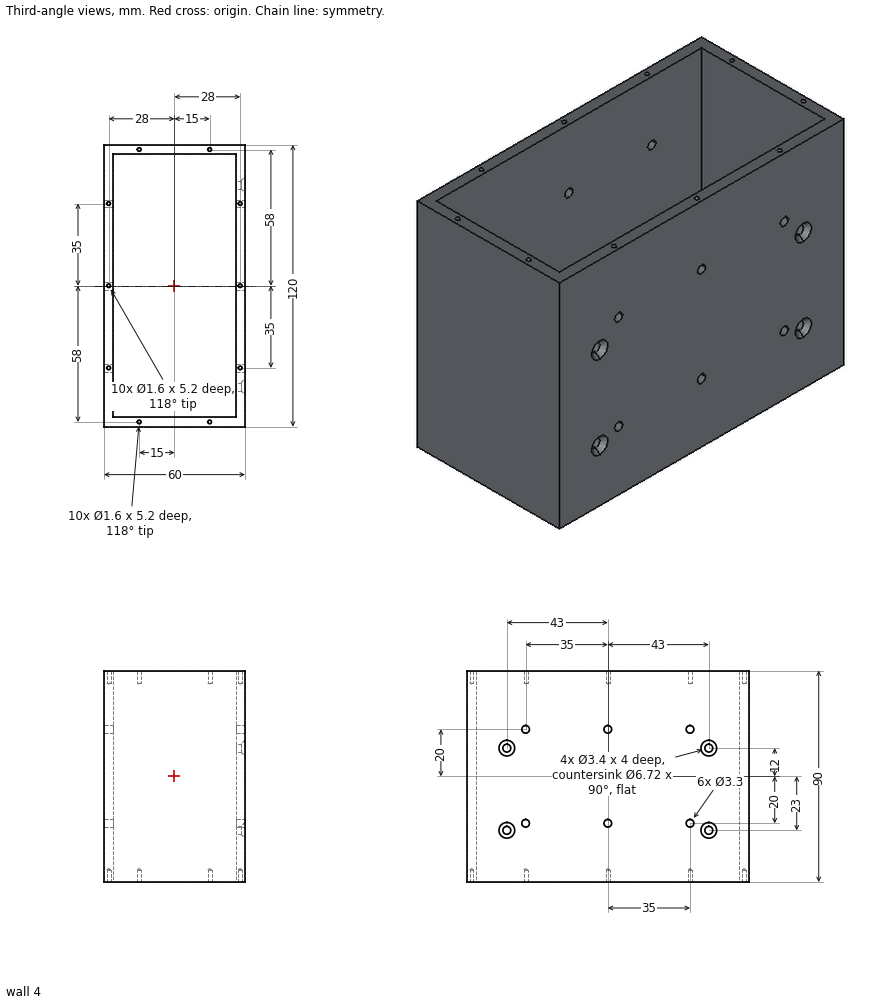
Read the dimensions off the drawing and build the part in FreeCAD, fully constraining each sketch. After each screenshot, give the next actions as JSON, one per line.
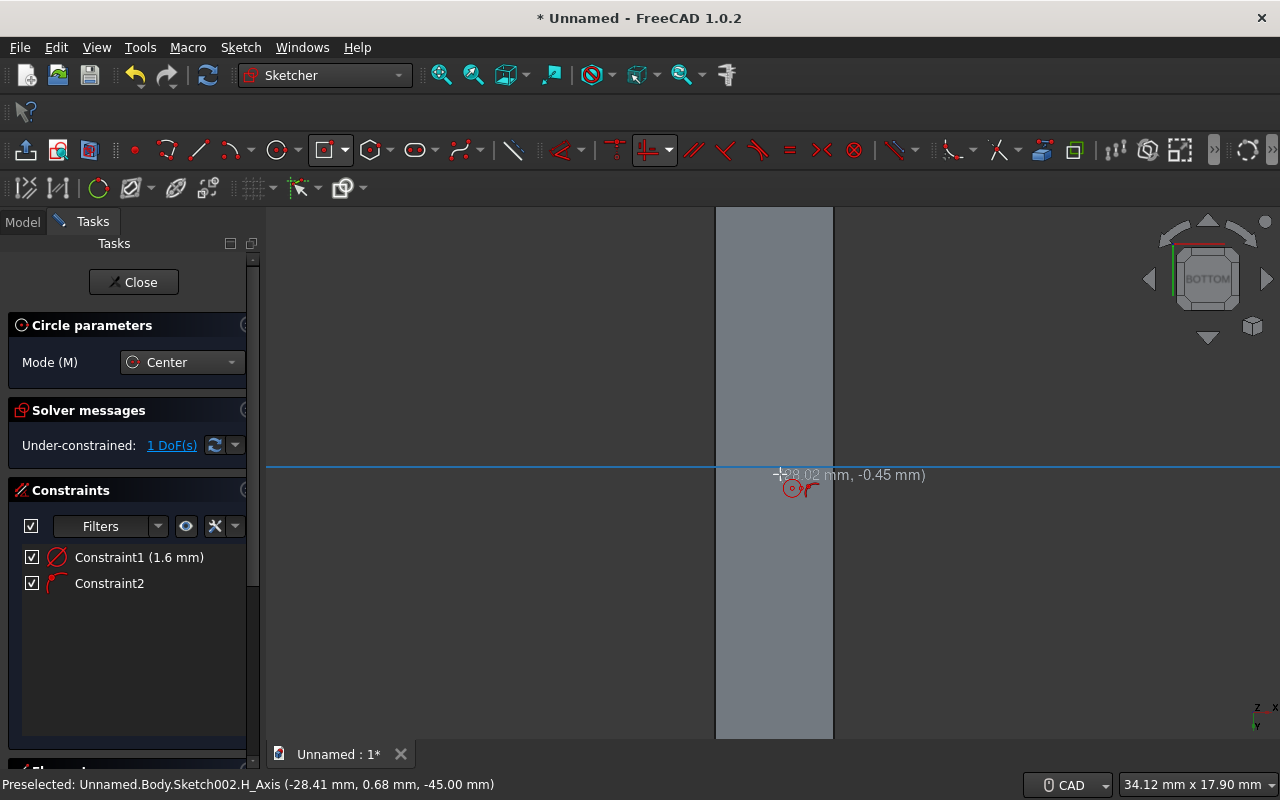
{"action": "scroll", "coordinate": [781, 474], "scroll_direction": "down", "scroll_amount": 12}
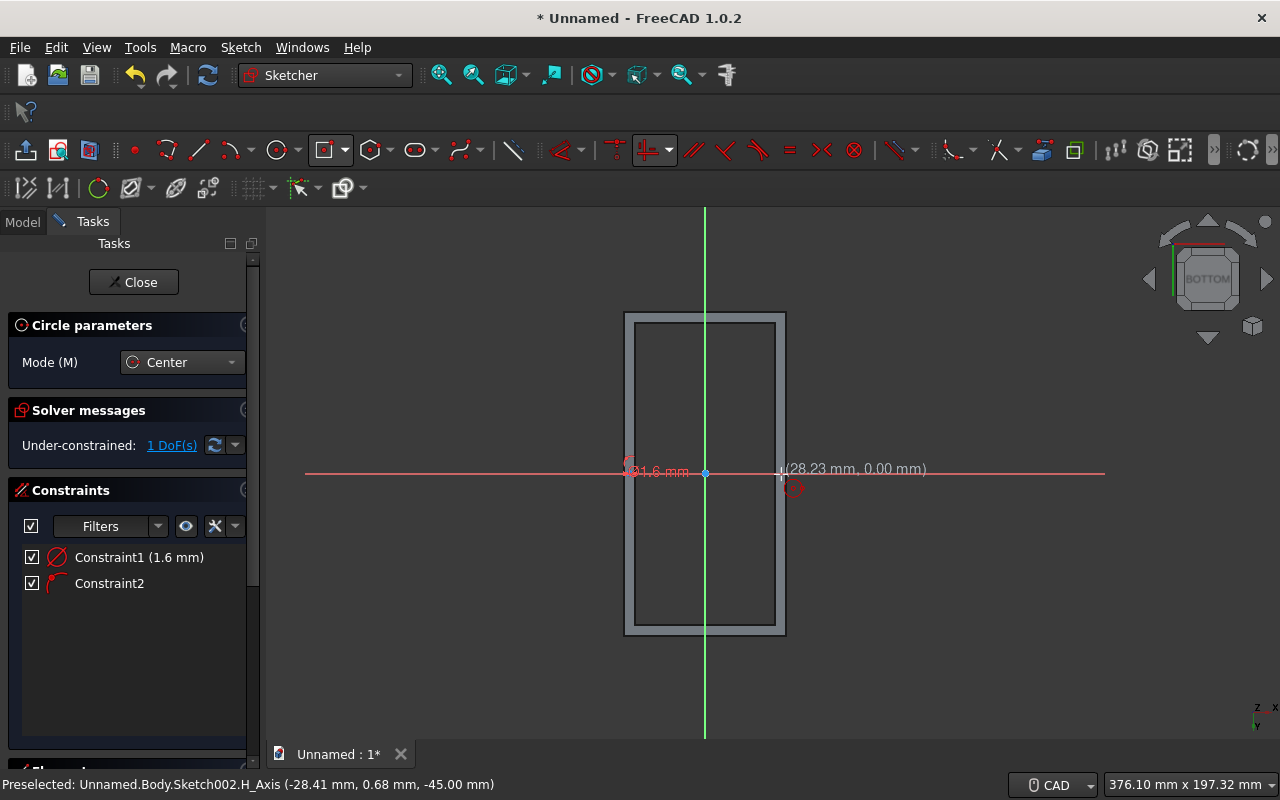
{"action": "left_click", "coordinate": [781, 474]}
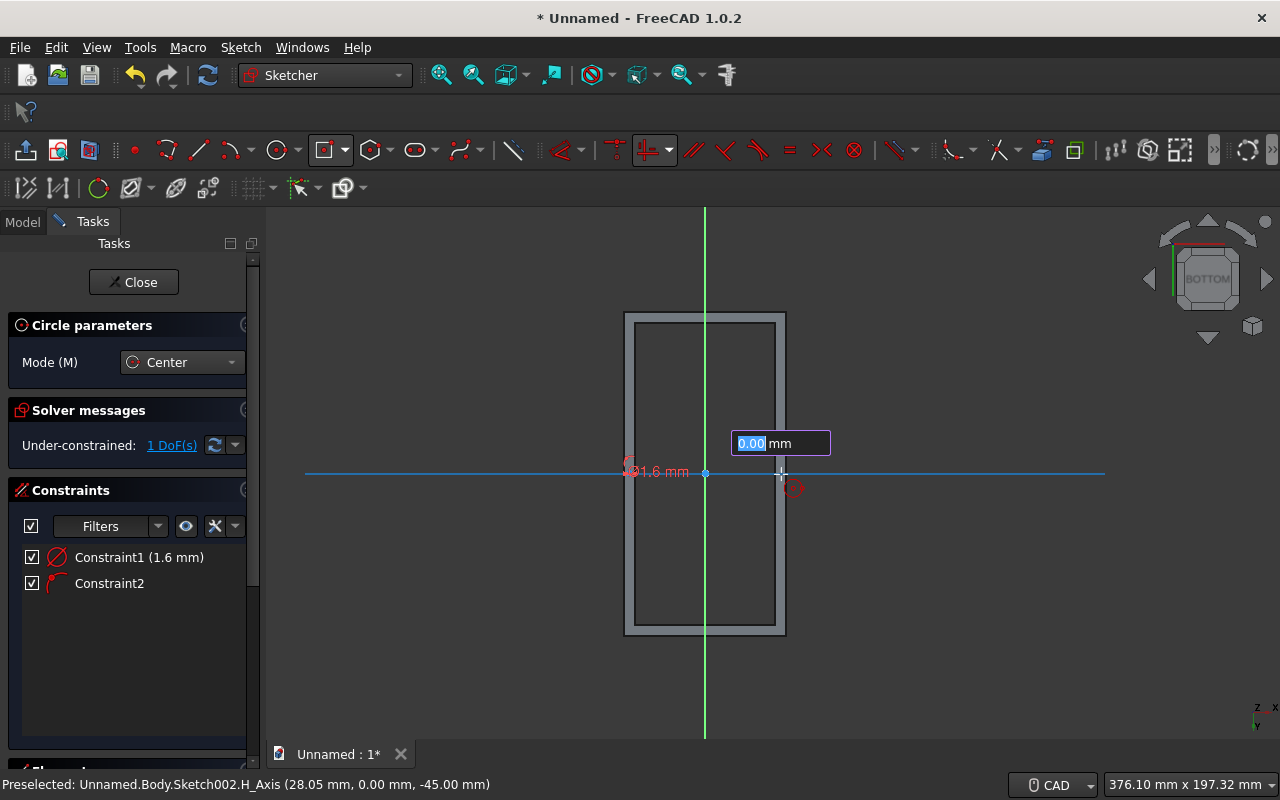
{"action": "scroll", "coordinate": [780, 476], "scroll_direction": "up", "scroll_amount": 11}
{"action": "mouse_move", "coordinate": [777, 470]}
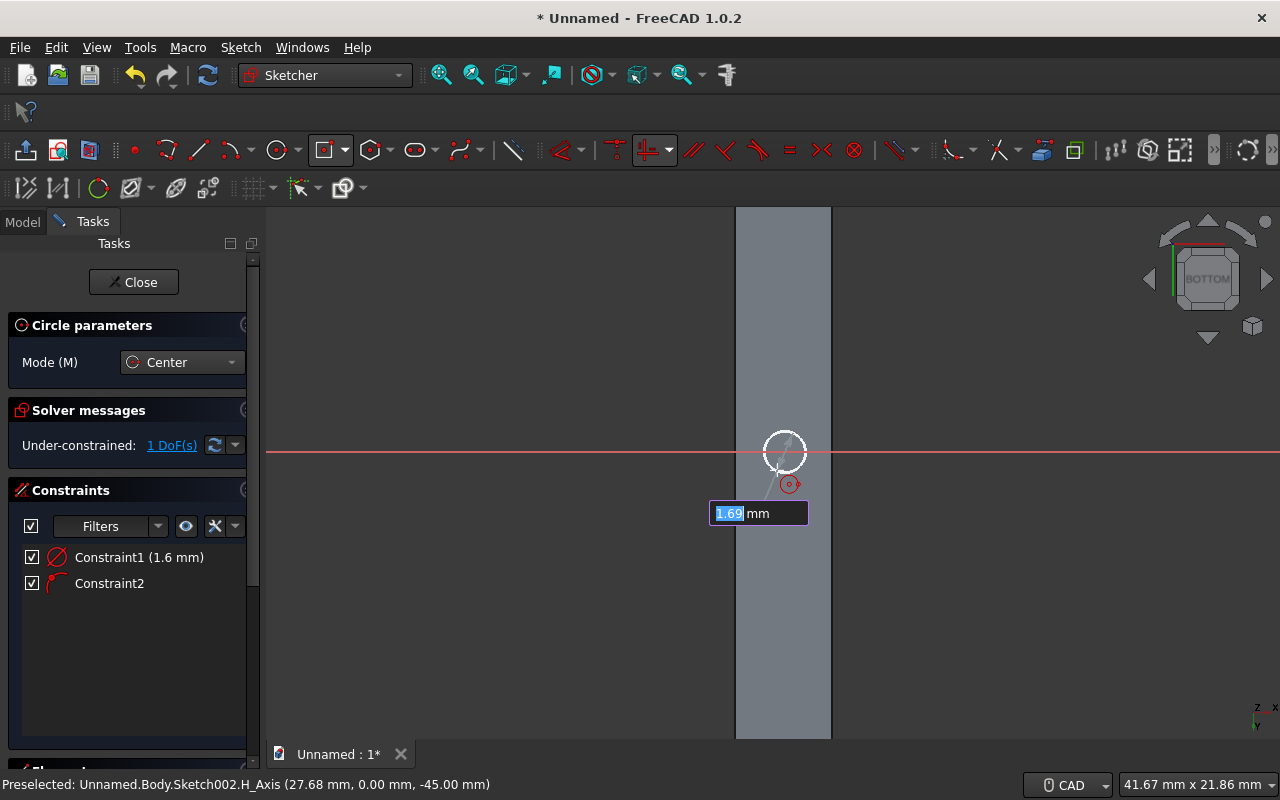
{"action": "type", "text": "1.6"}
{"action": "key", "text": "Return"}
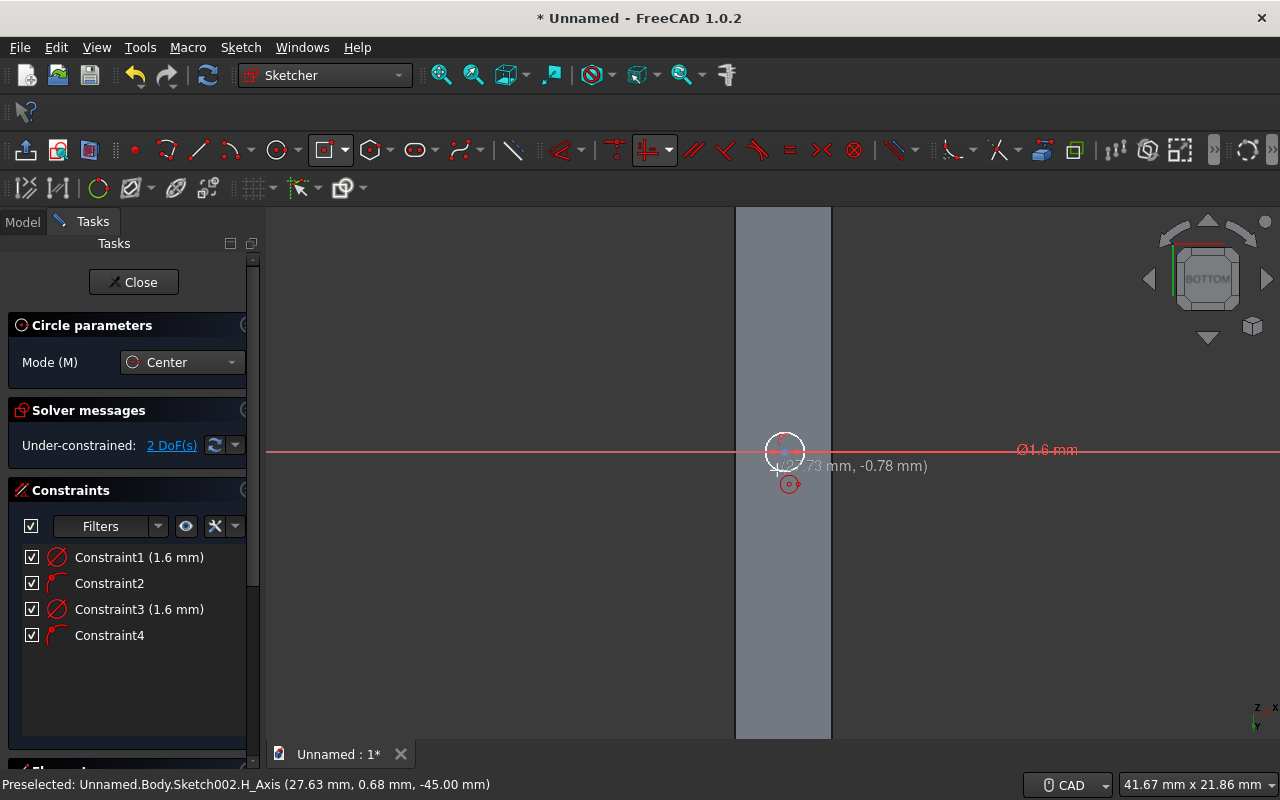
{"action": "scroll", "coordinate": [780, 476], "scroll_direction": "down", "scroll_amount": 11}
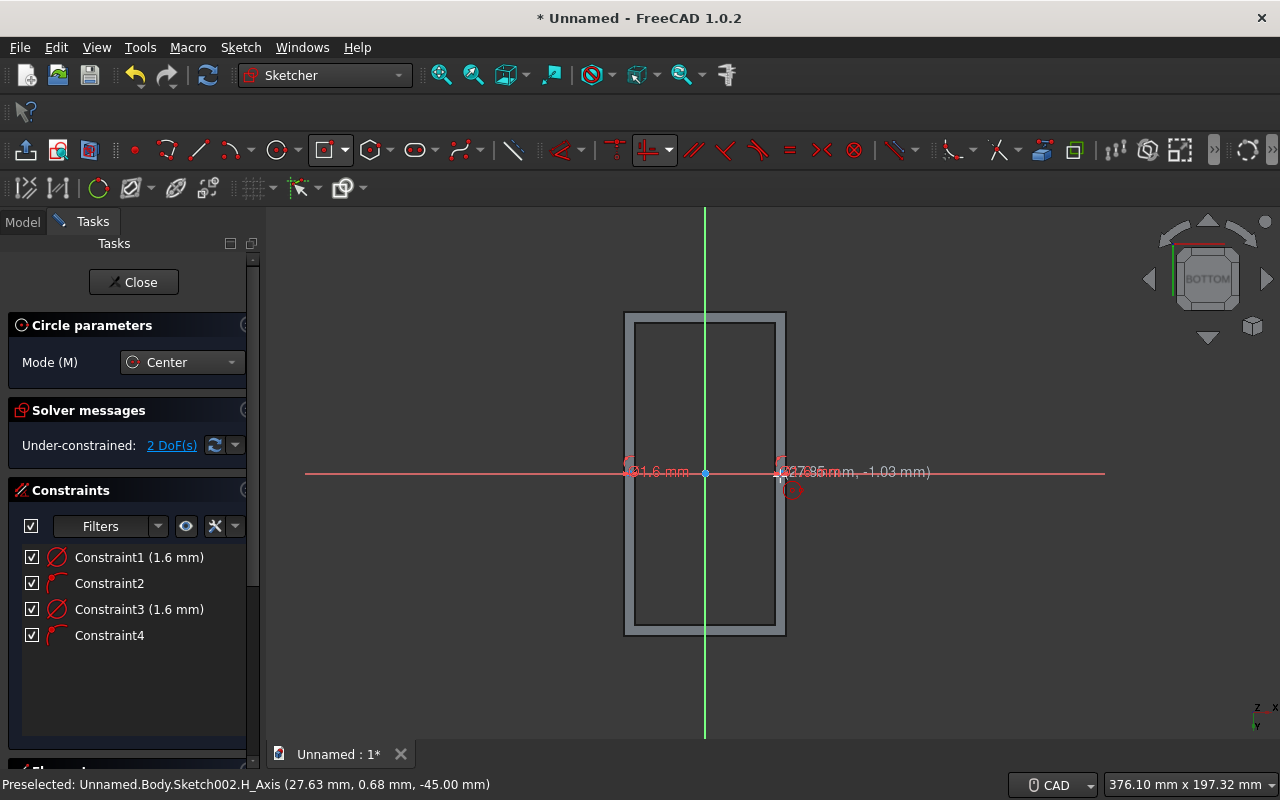
{"action": "scroll", "coordinate": [746, 630], "scroll_direction": "up", "scroll_amount": 12}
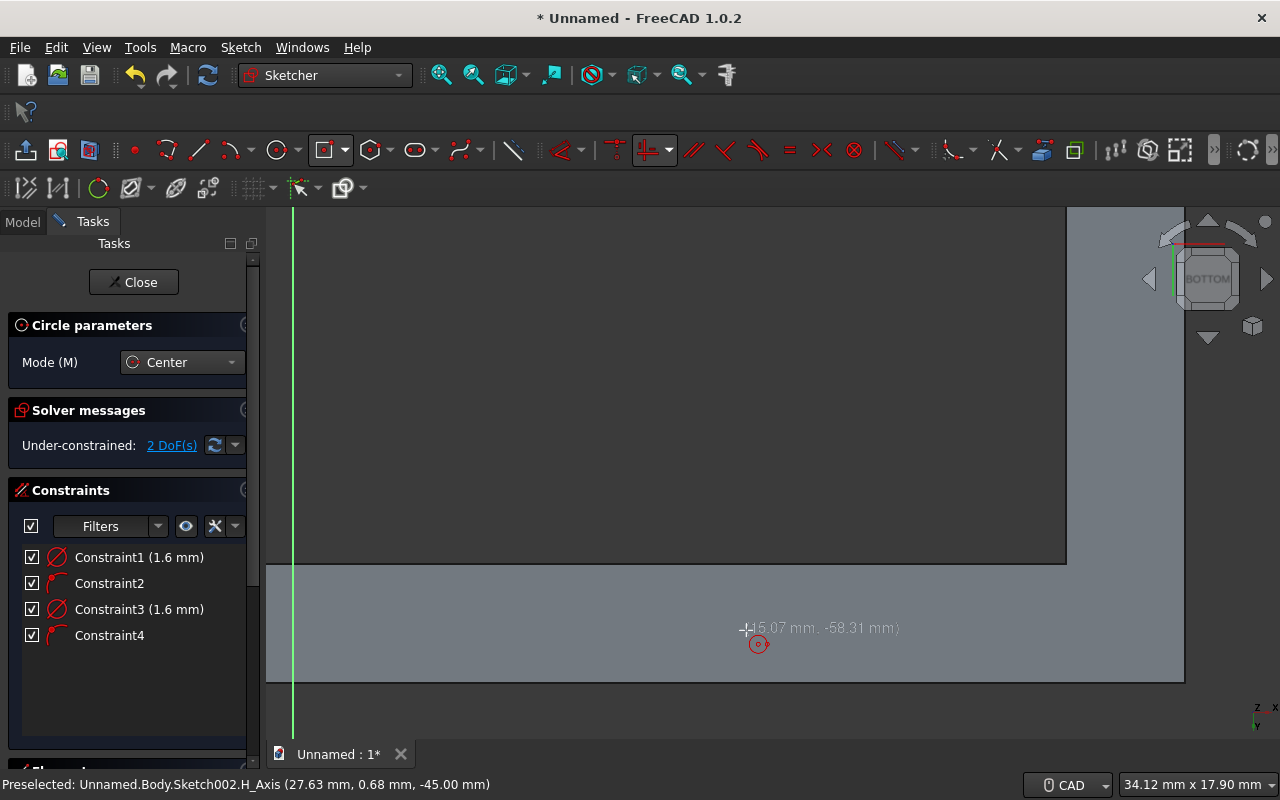
{"action": "scroll", "coordinate": [746, 630], "scroll_direction": "down", "scroll_amount": 12}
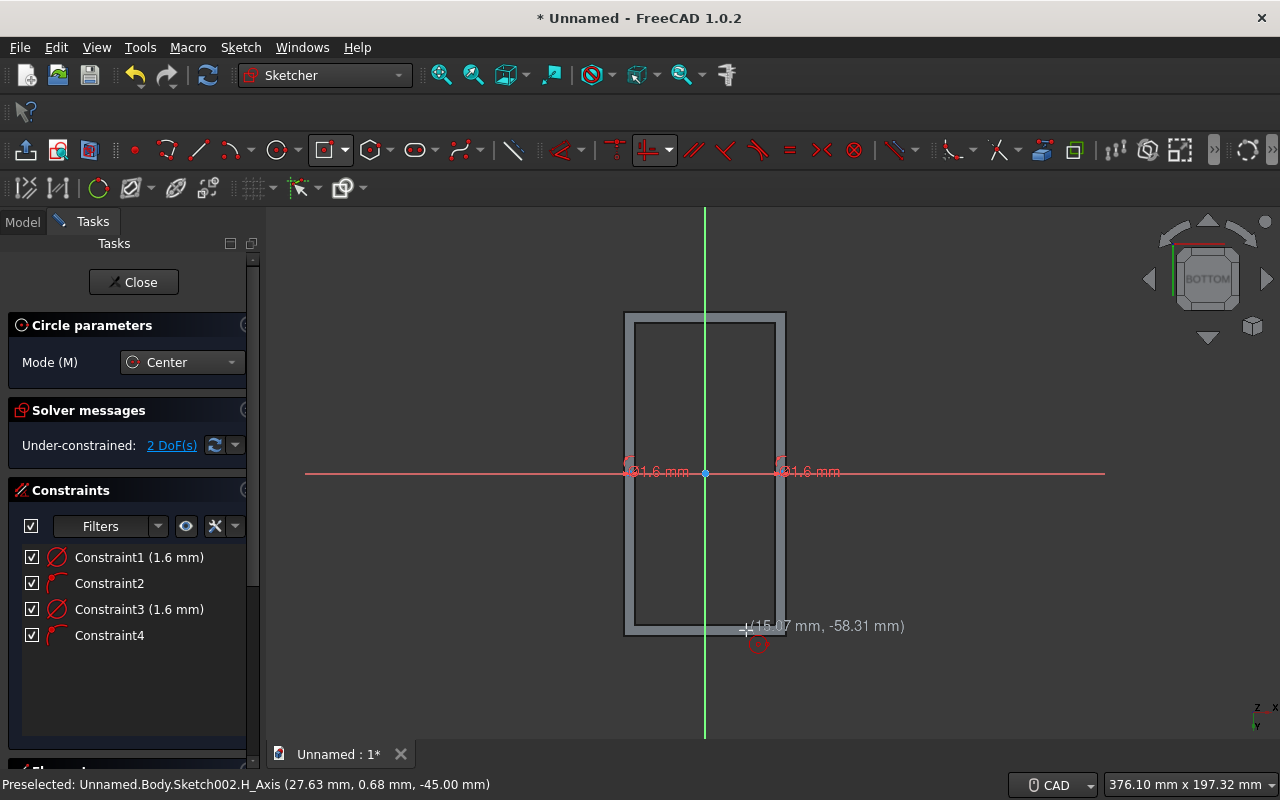
{"action": "left_click", "coordinate": [746, 630]}
{"action": "mouse_move", "coordinate": [747, 629]}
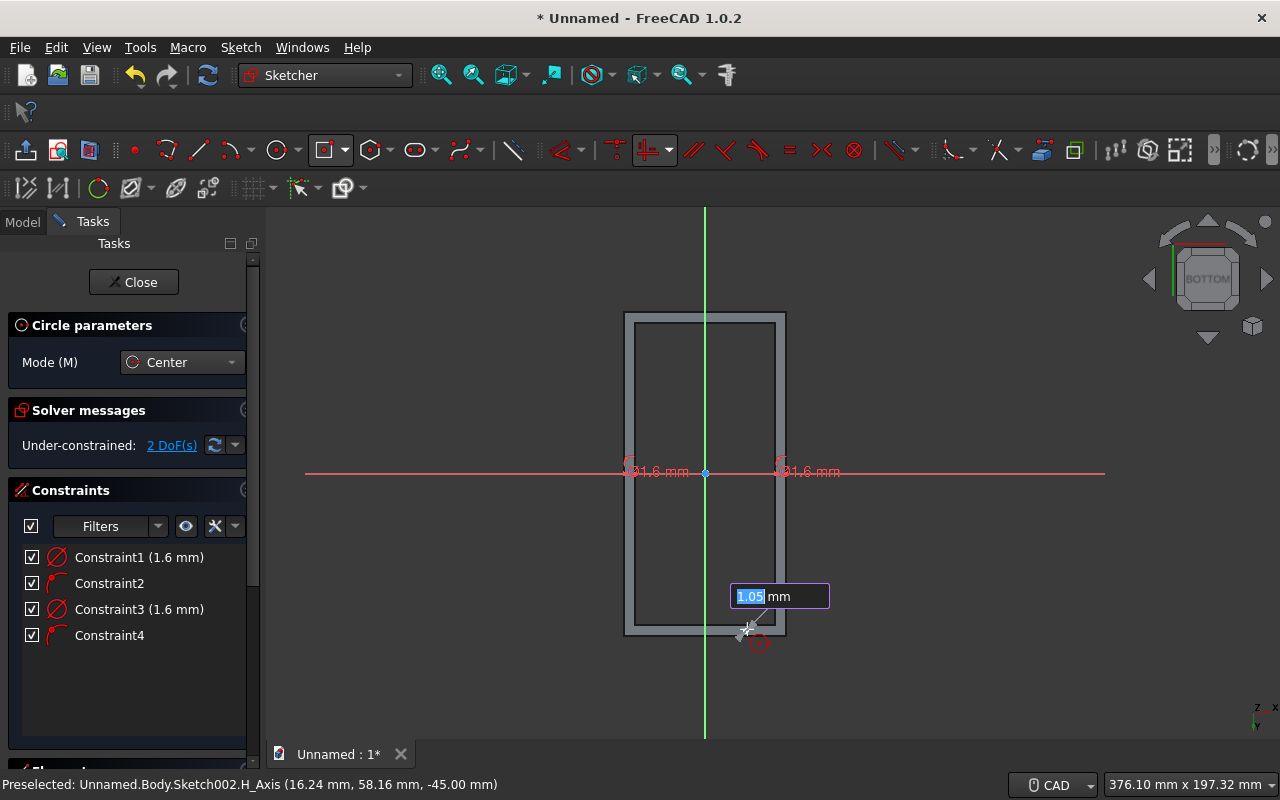
{"action": "type", "text": "1.6"}
{"action": "key", "text": "Return"}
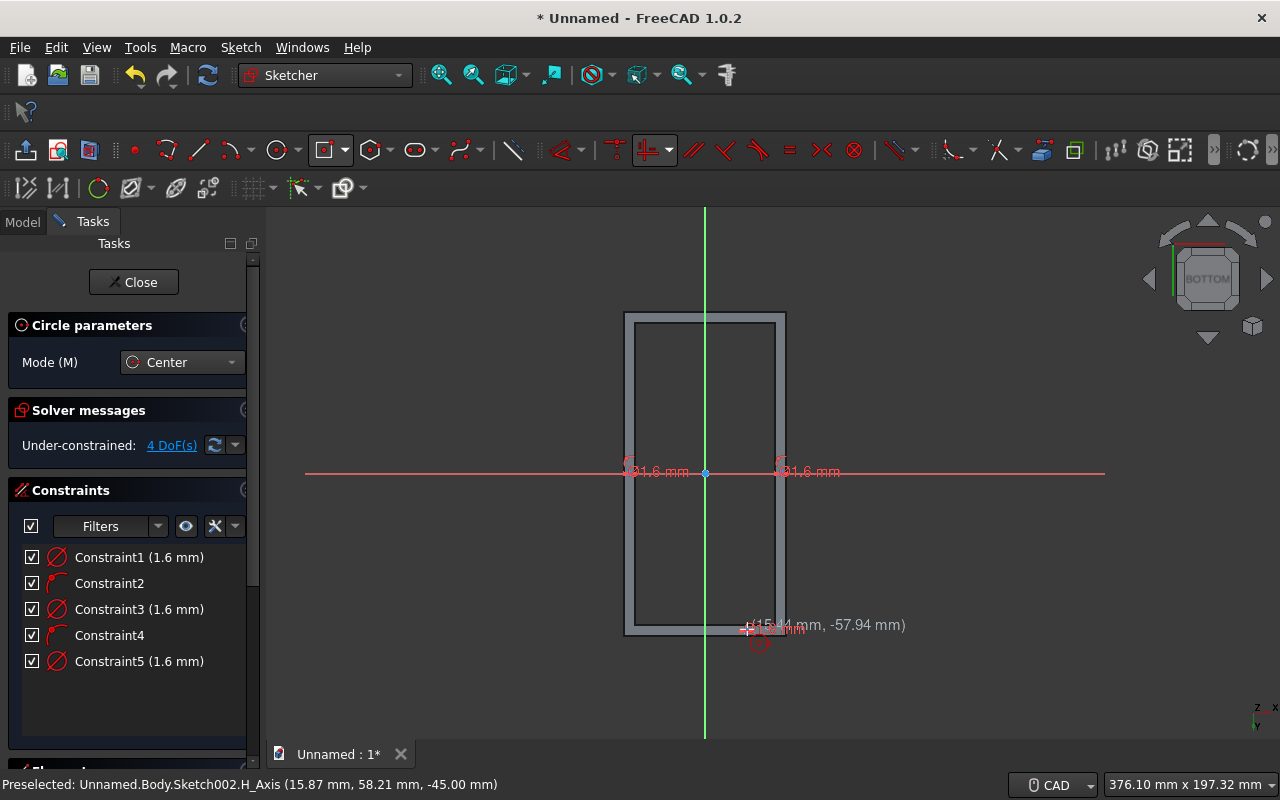
{"action": "scroll", "coordinate": [665, 630], "scroll_direction": "up", "scroll_amount": 12}